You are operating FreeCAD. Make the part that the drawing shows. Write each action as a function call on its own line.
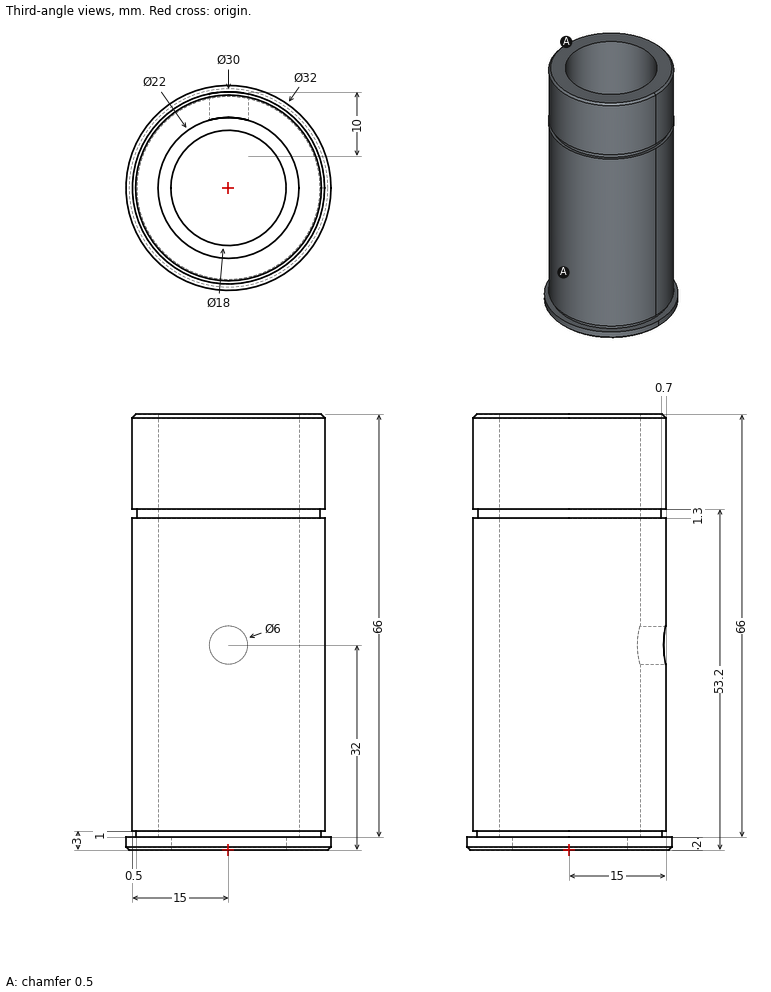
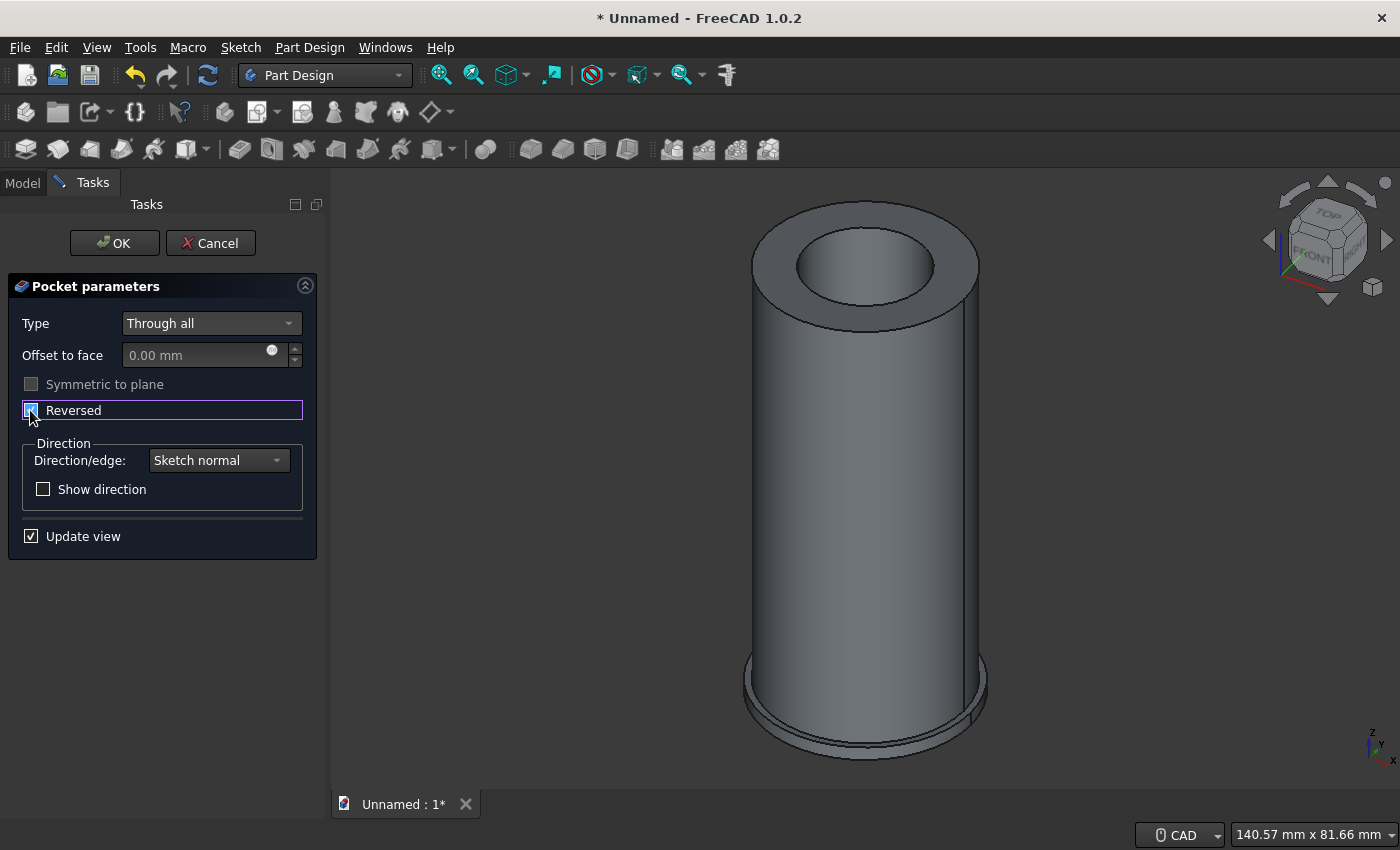
click(115, 243)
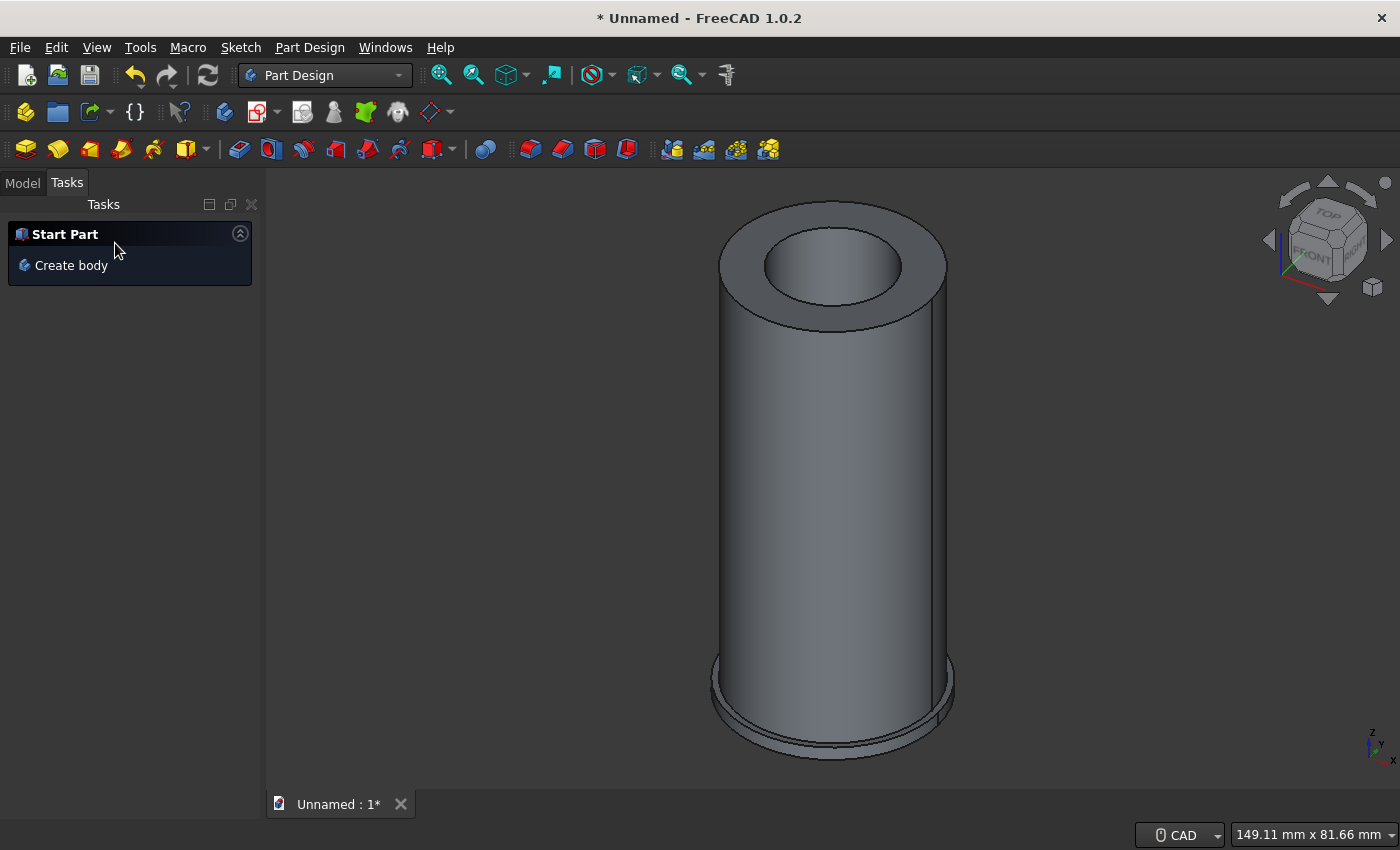
click(744, 279)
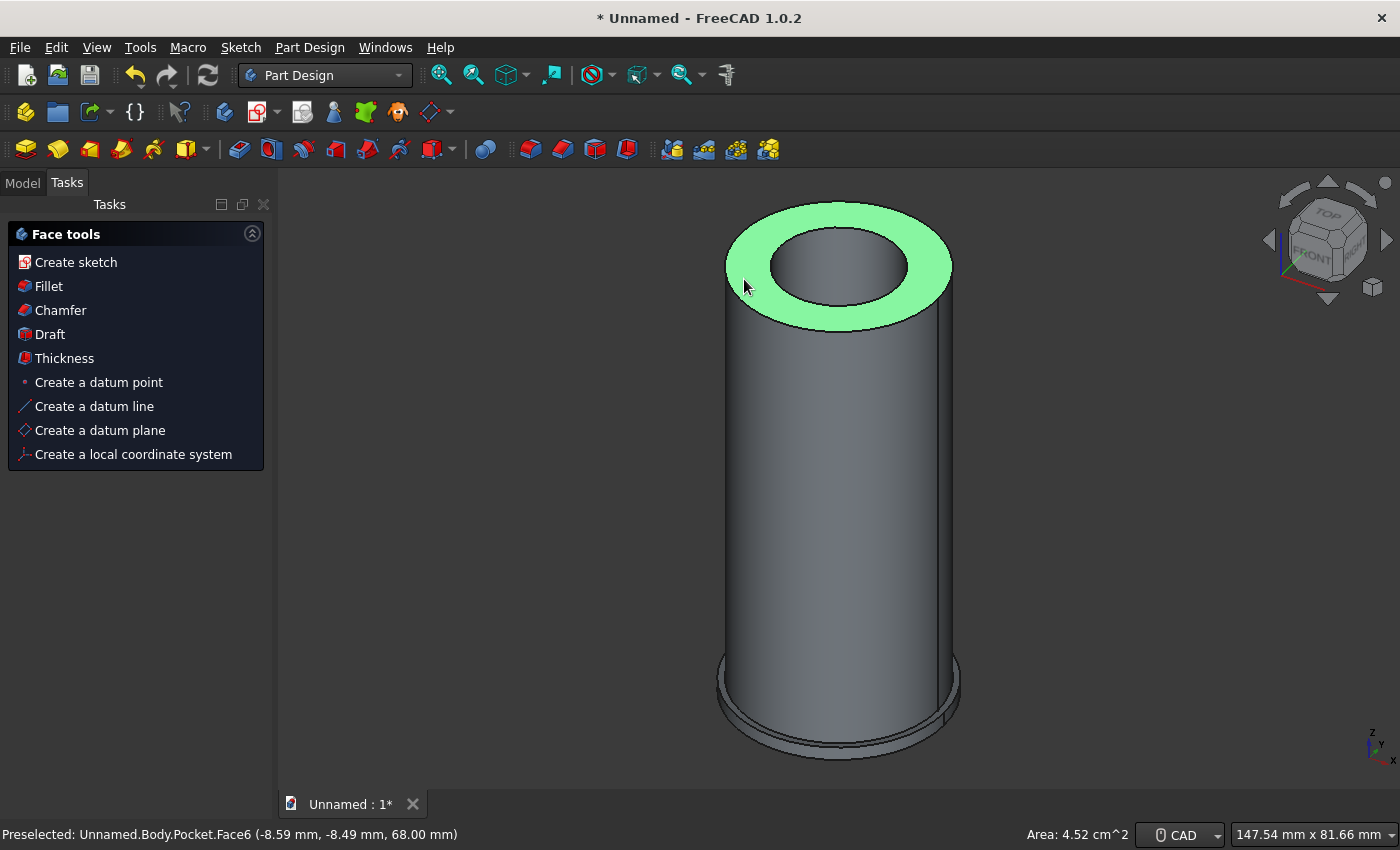
click(258, 112)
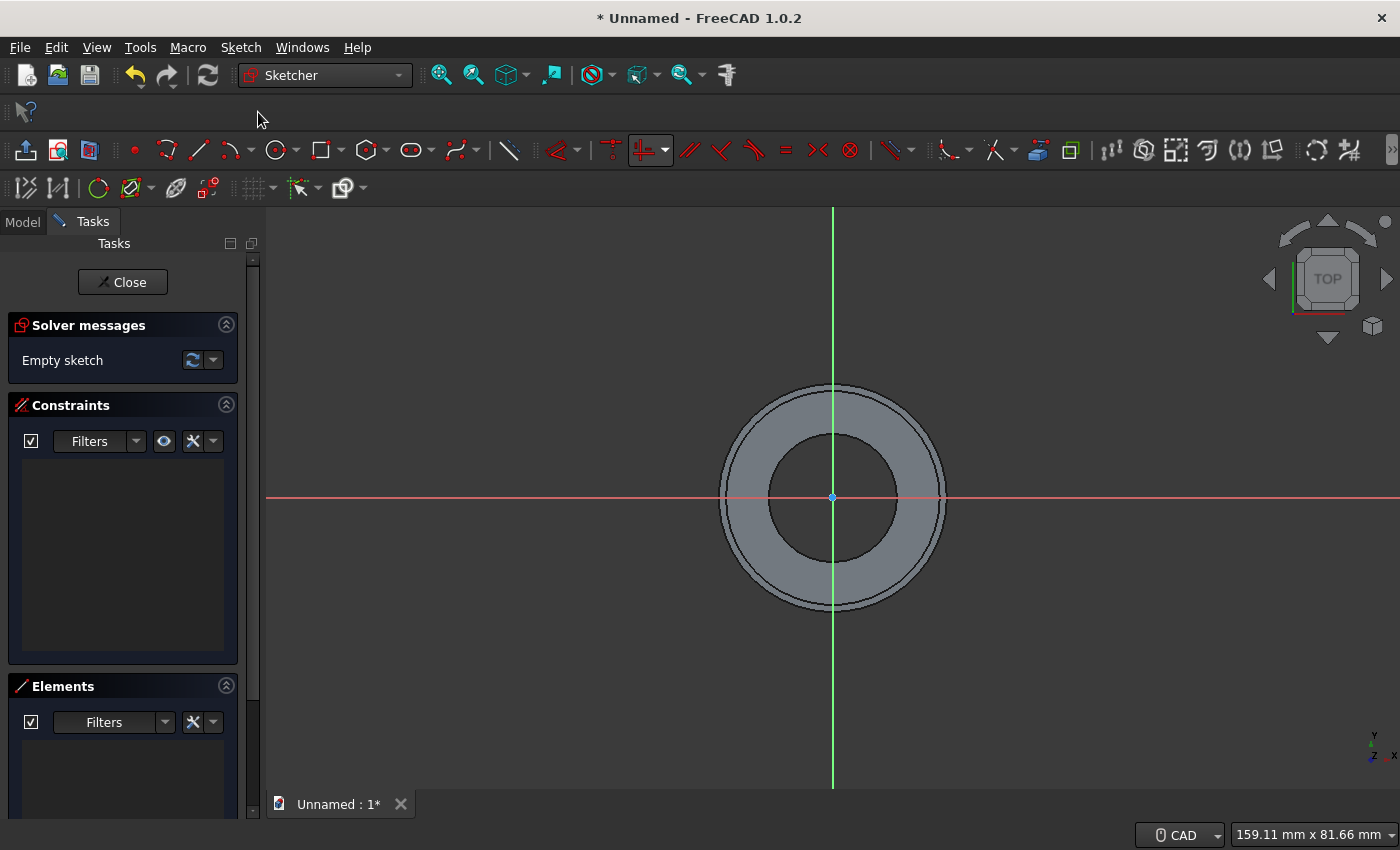
scroll(889, 498, up, 4)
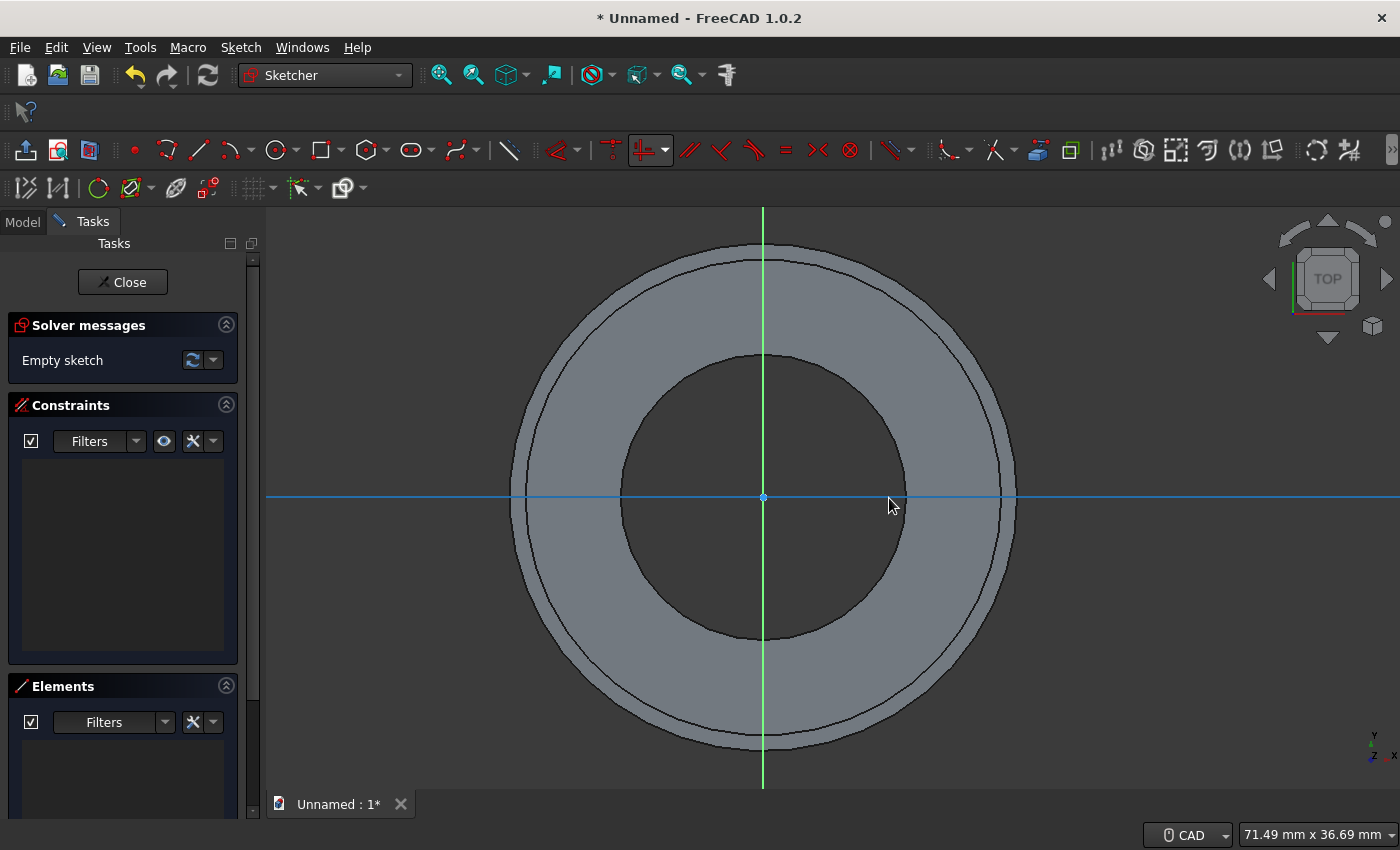
click(276, 150)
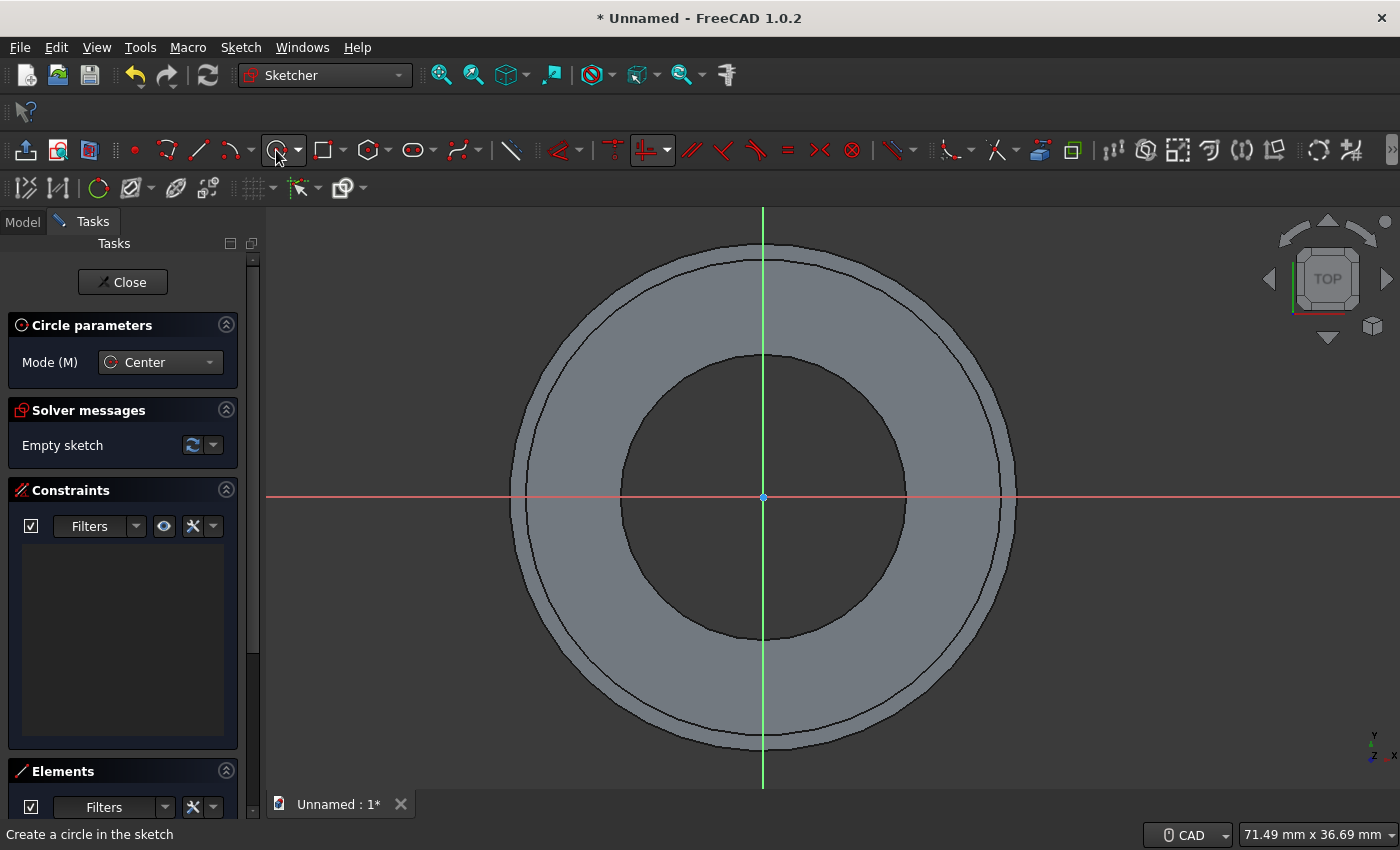
click(763, 497)
move(887, 374)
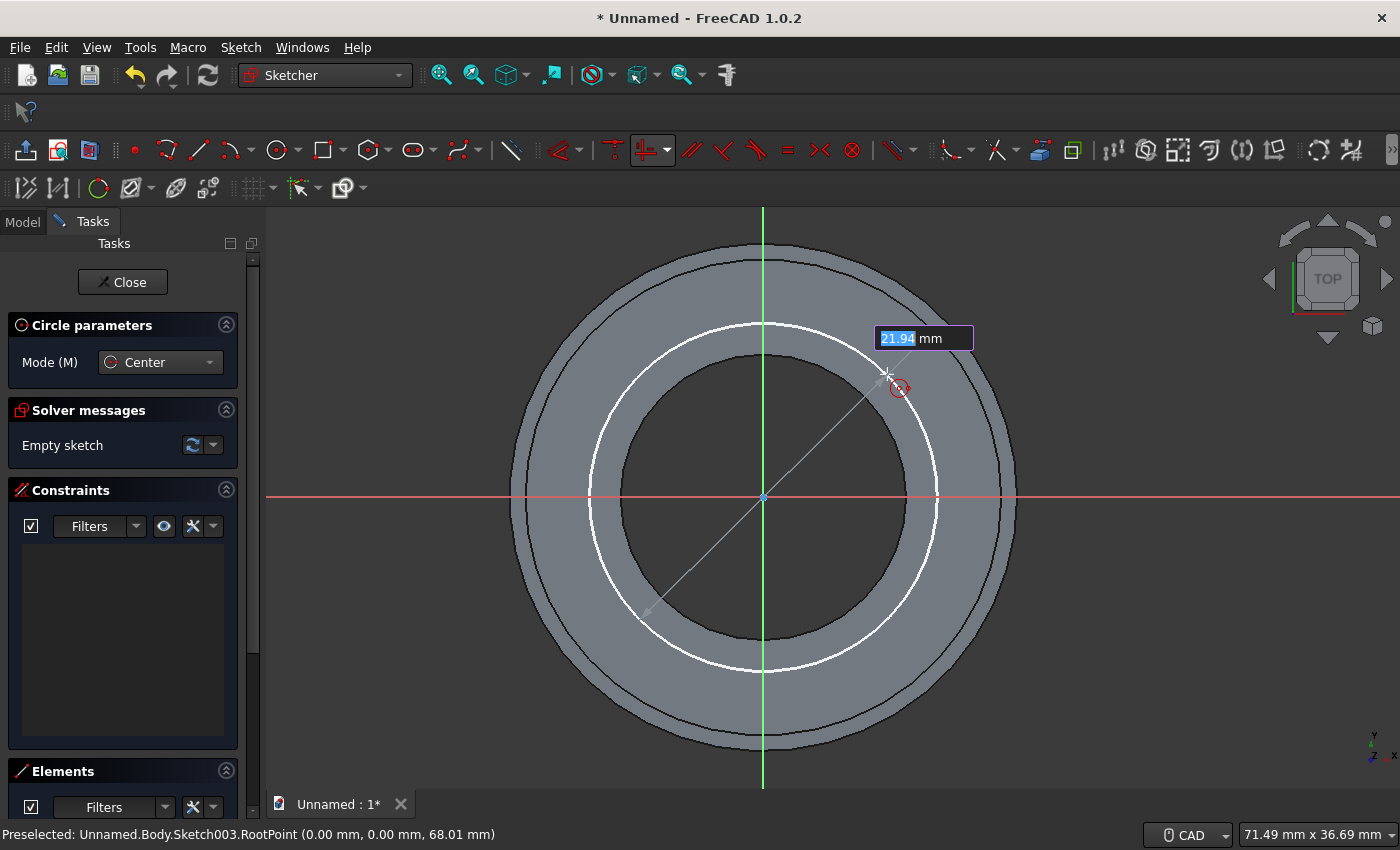
text(22)
key(Return)
key(Escape)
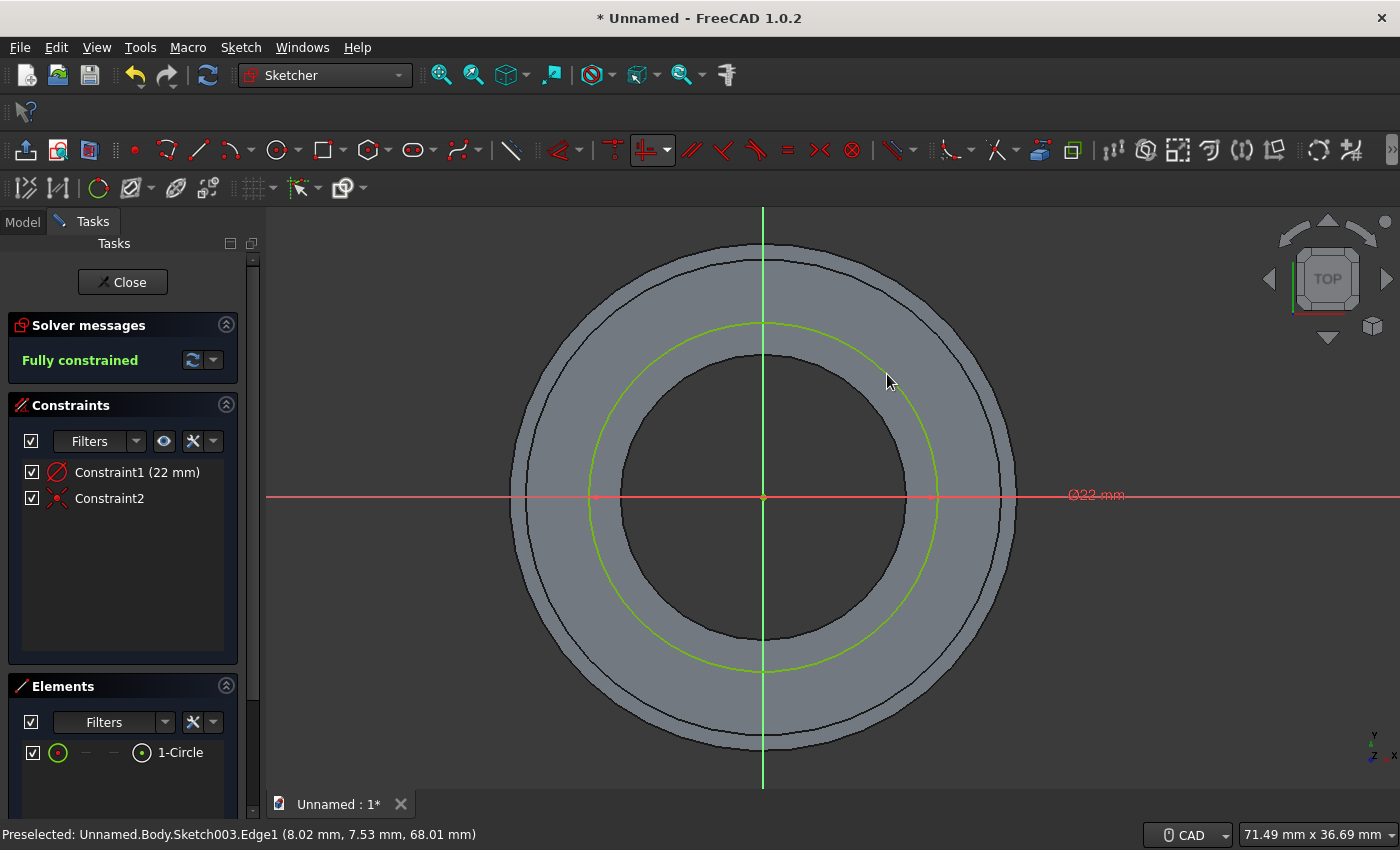
click(123, 282)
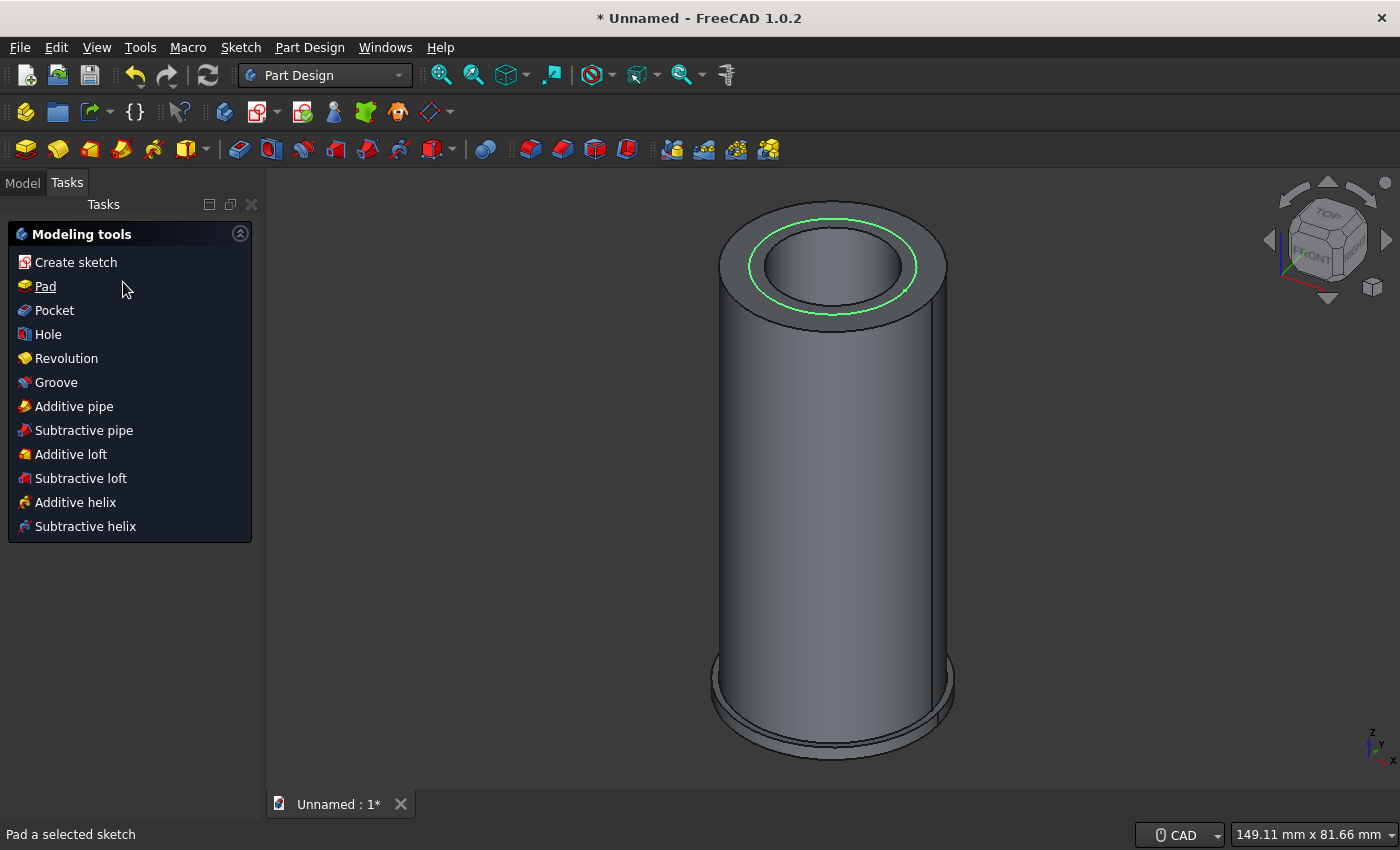
click(240, 150)